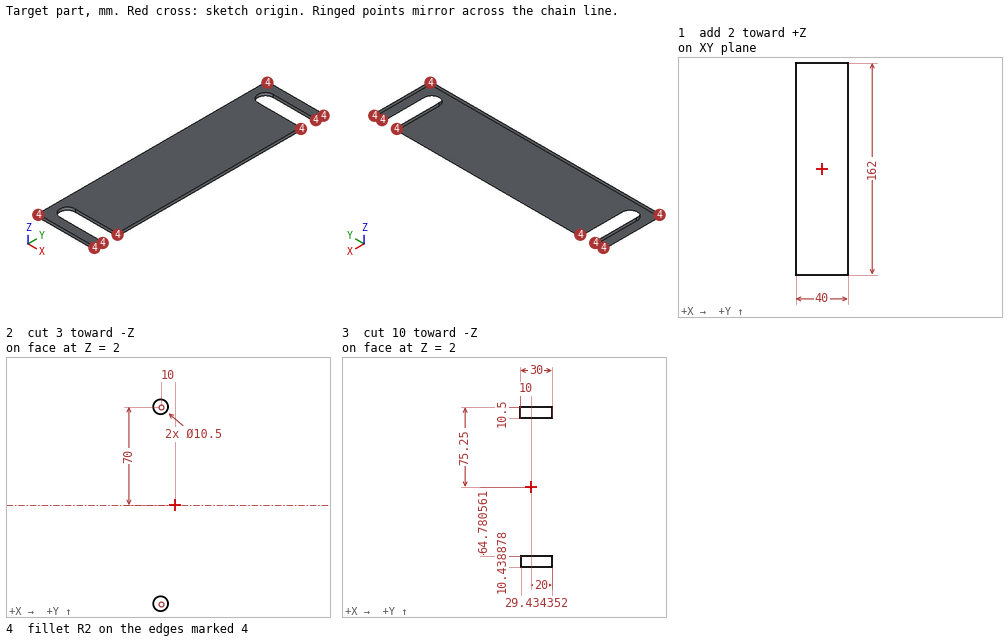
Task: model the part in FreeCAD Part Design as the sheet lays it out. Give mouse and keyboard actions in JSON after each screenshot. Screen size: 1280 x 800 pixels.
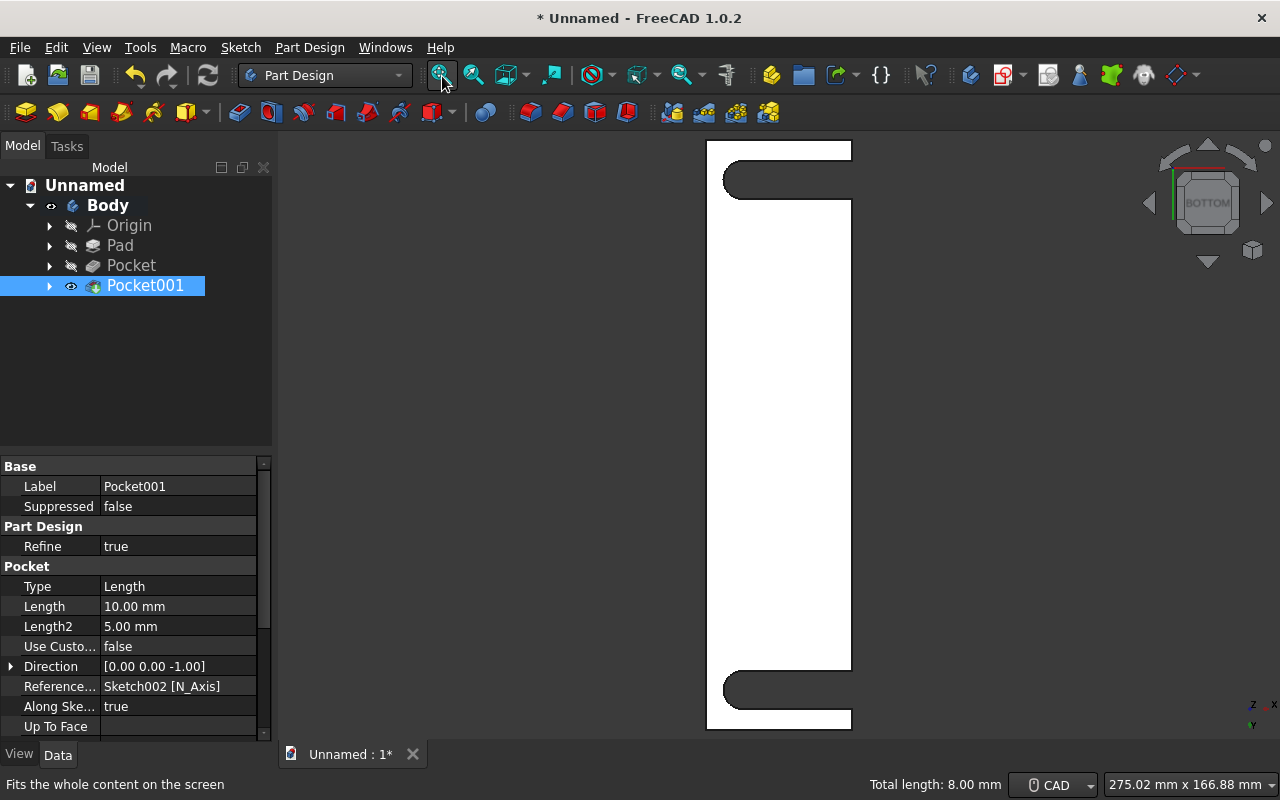
{"action": "key", "text": "4"}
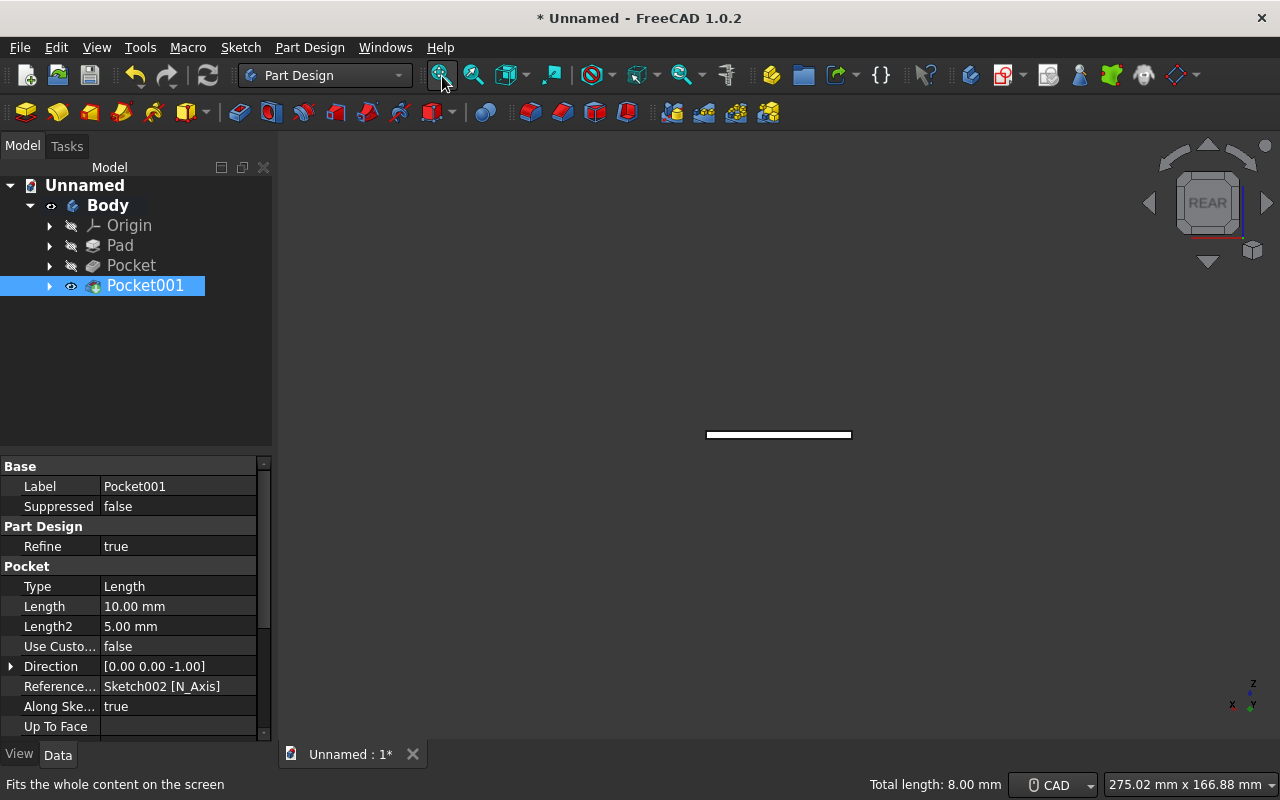
{"action": "left_click", "coordinate": [442, 76]}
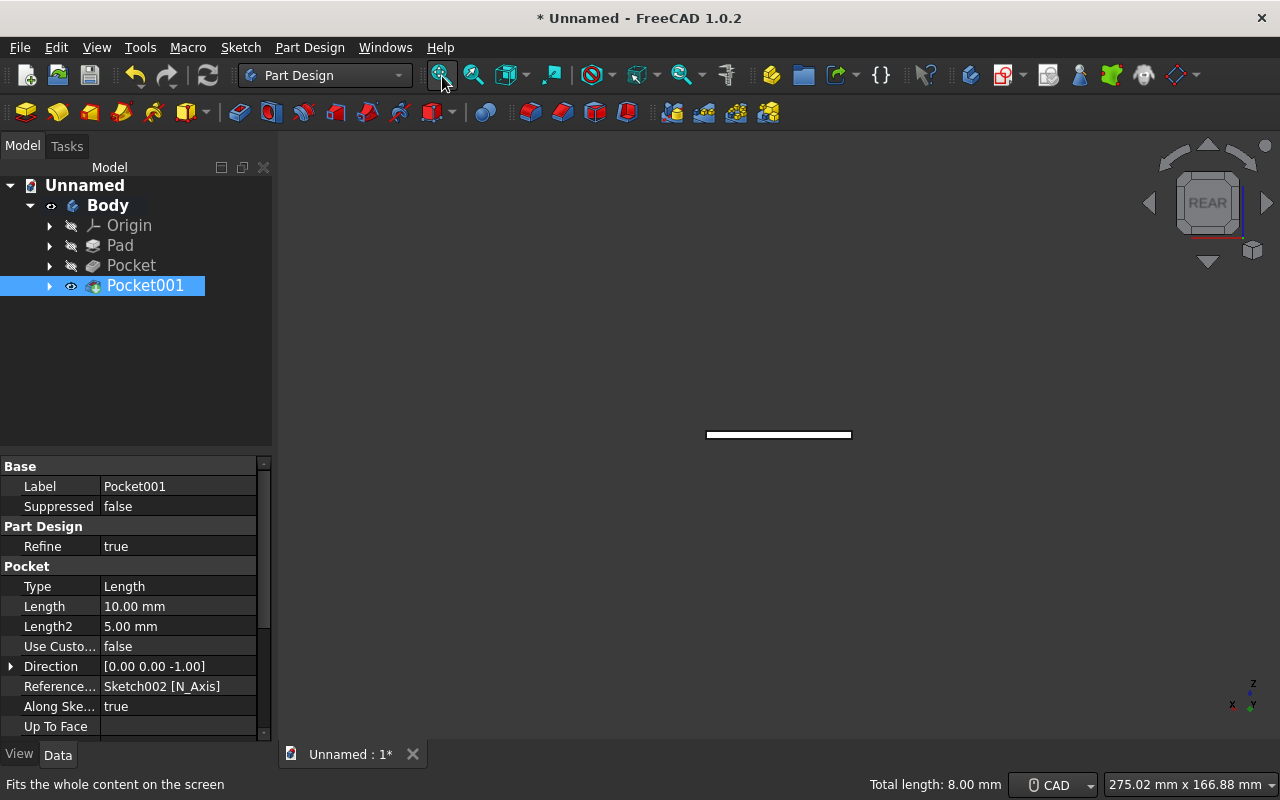
{"action": "scroll", "coordinate": [706, 434], "scroll_direction": "up", "scroll_amount": 9}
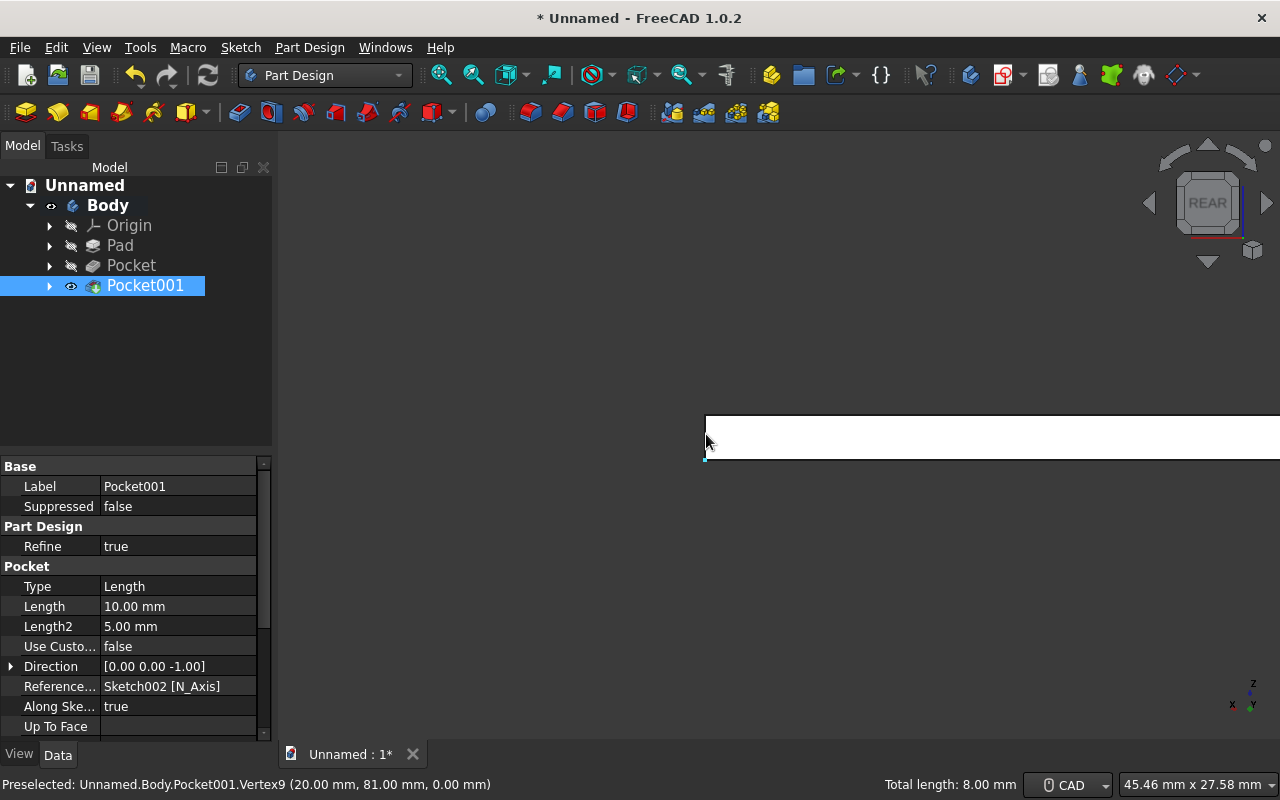
{"action": "left_click", "coordinate": [705, 437], "text": "ctrl"}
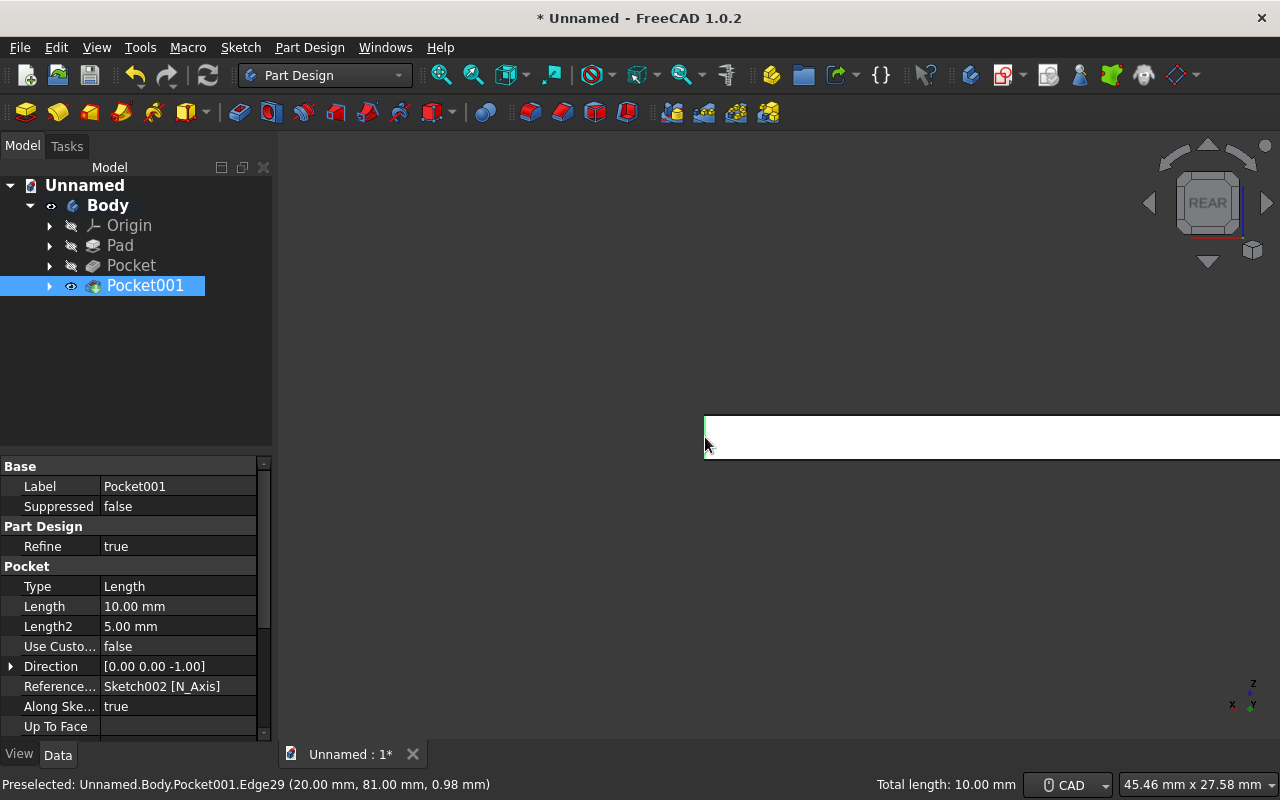
{"action": "key", "text": "v f"}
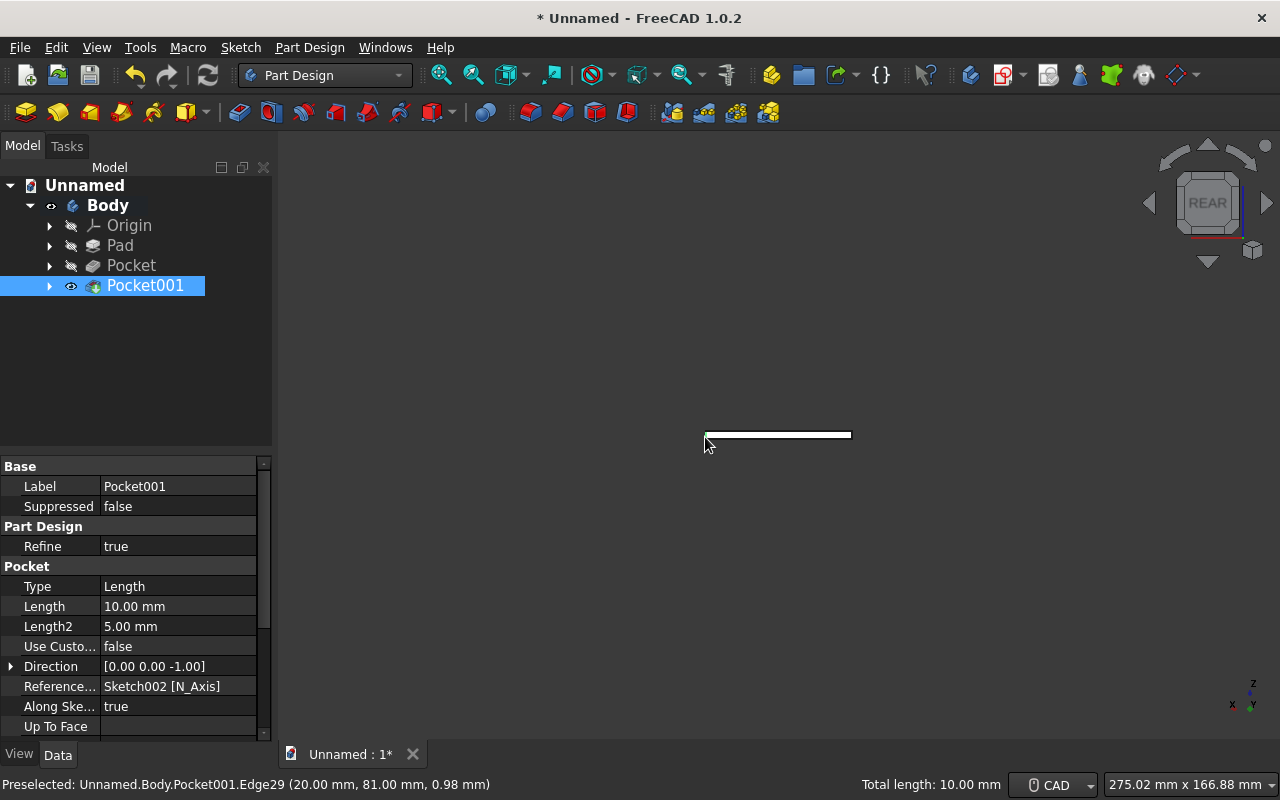
{"action": "key", "text": "6"}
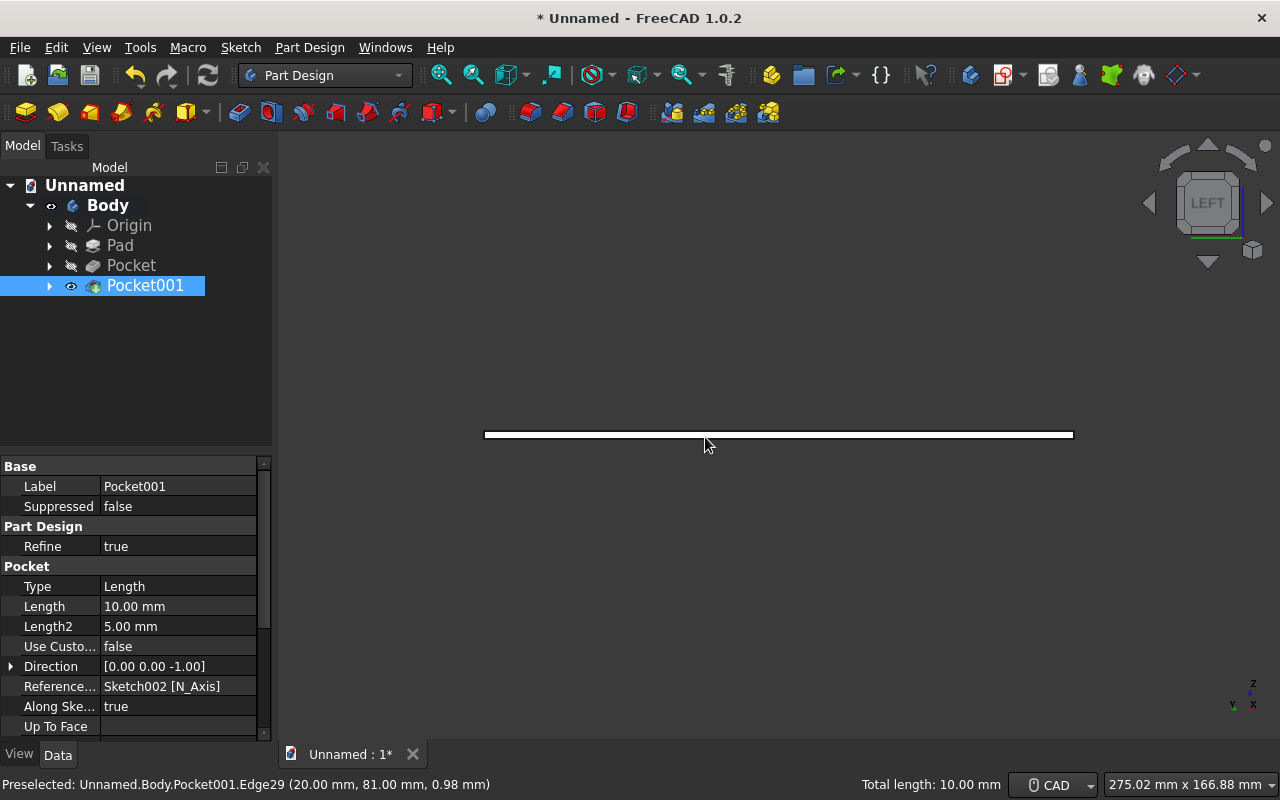
{"action": "scroll", "coordinate": [1053, 434], "scroll_direction": "up", "scroll_amount": 9}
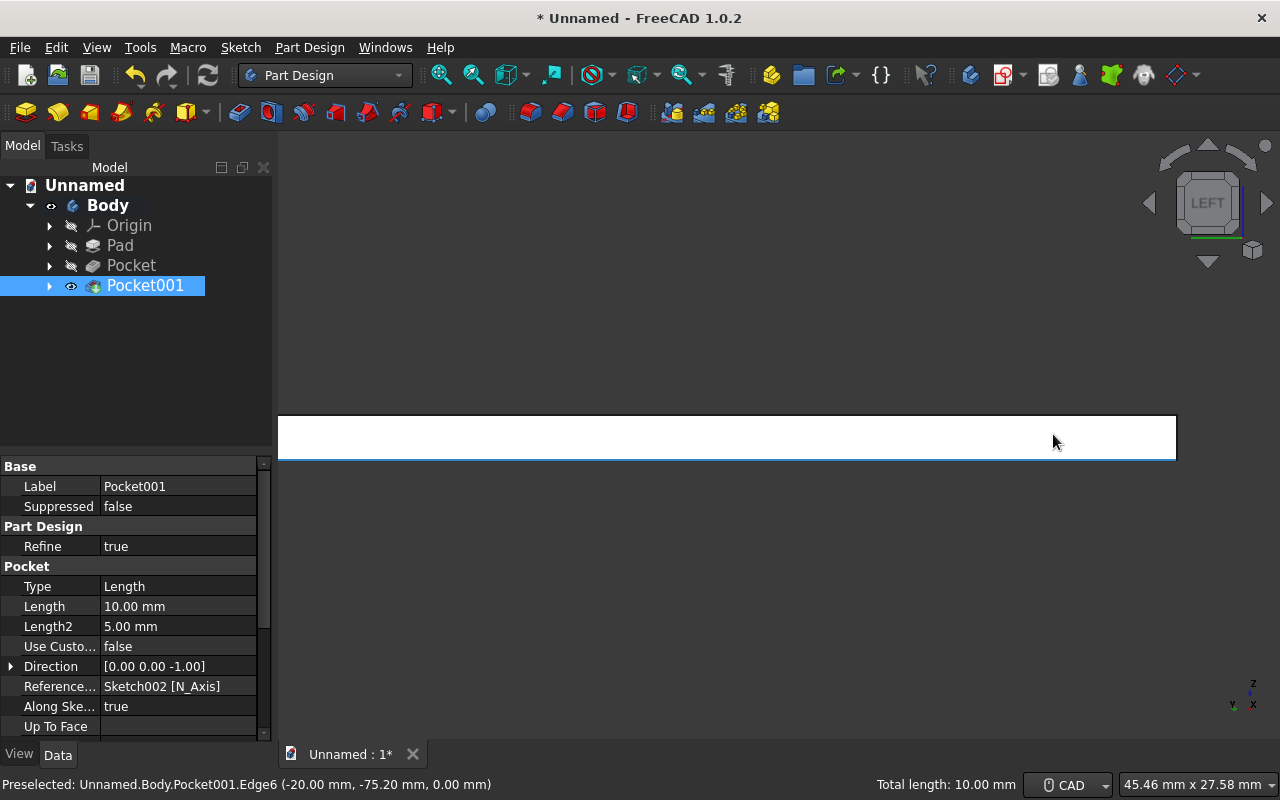
{"action": "left_click", "coordinate": [1177, 437], "text": "ctrl"}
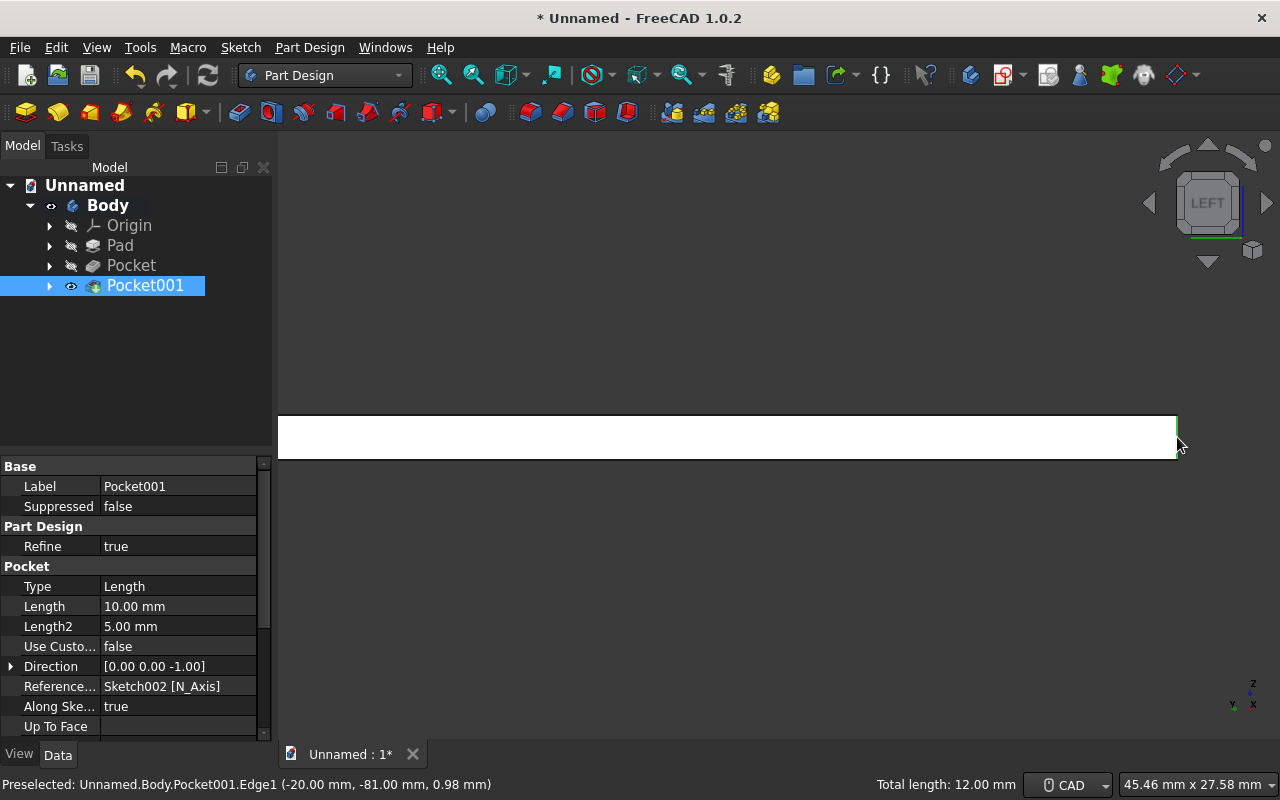
{"action": "key", "text": "v f"}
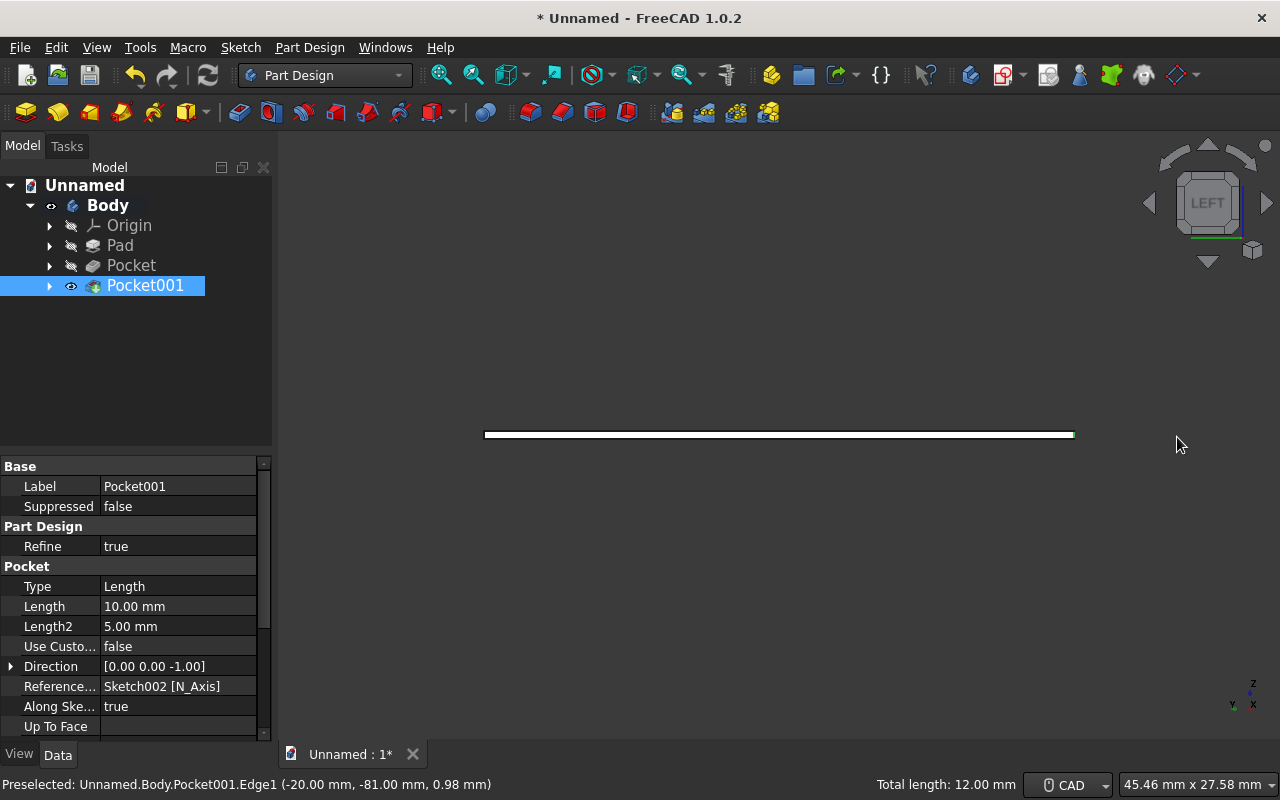
{"action": "key", "text": "v 3"}